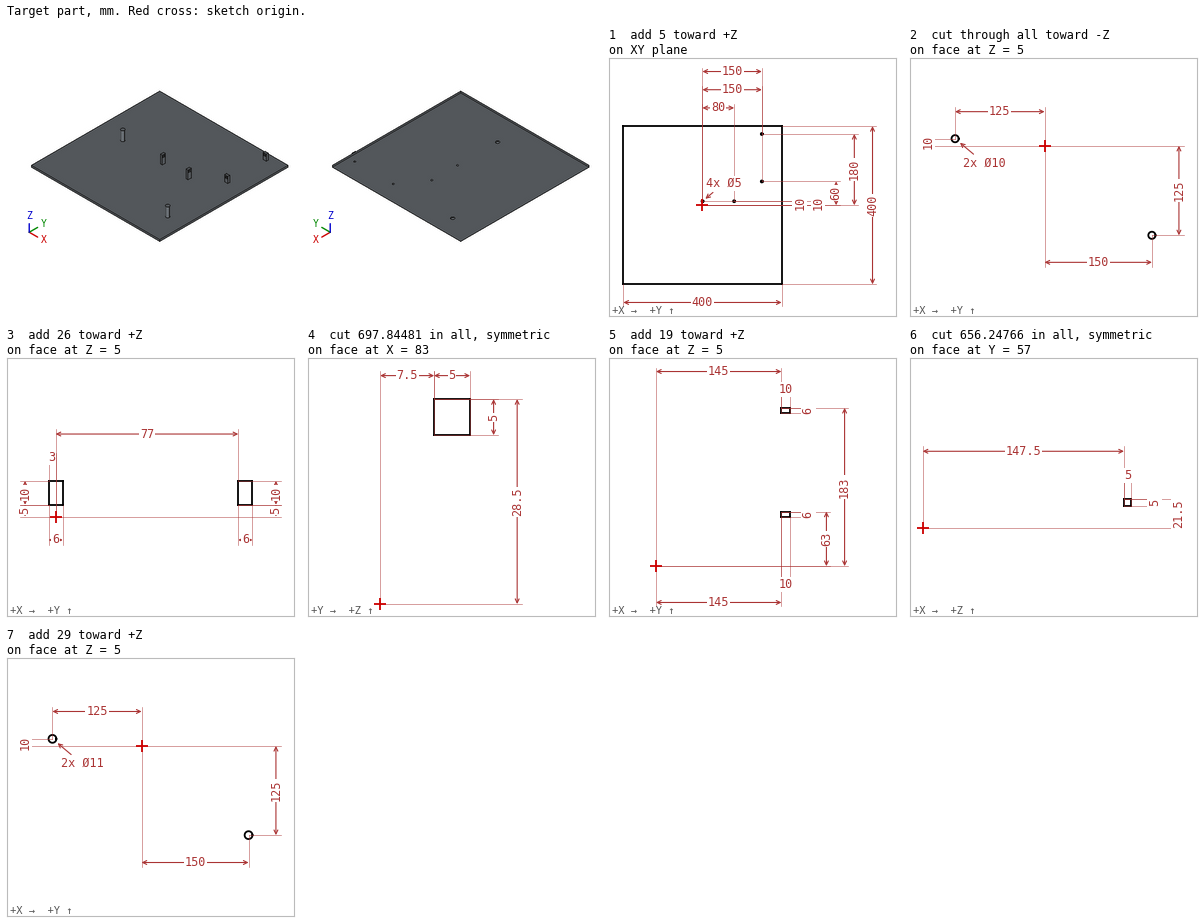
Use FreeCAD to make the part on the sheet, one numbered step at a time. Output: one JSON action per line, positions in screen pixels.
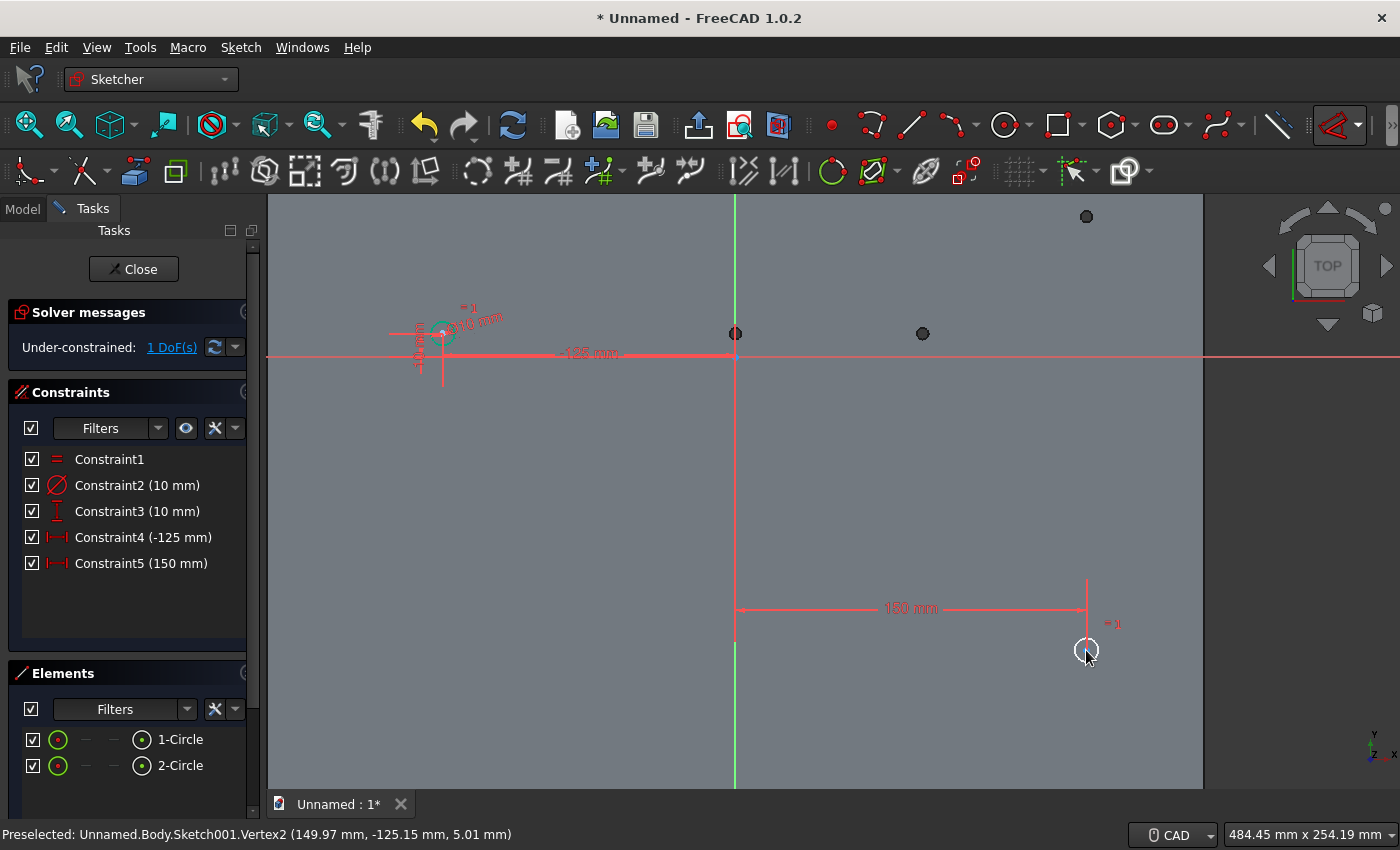
{"action": "left_click", "coordinate": [1087, 650]}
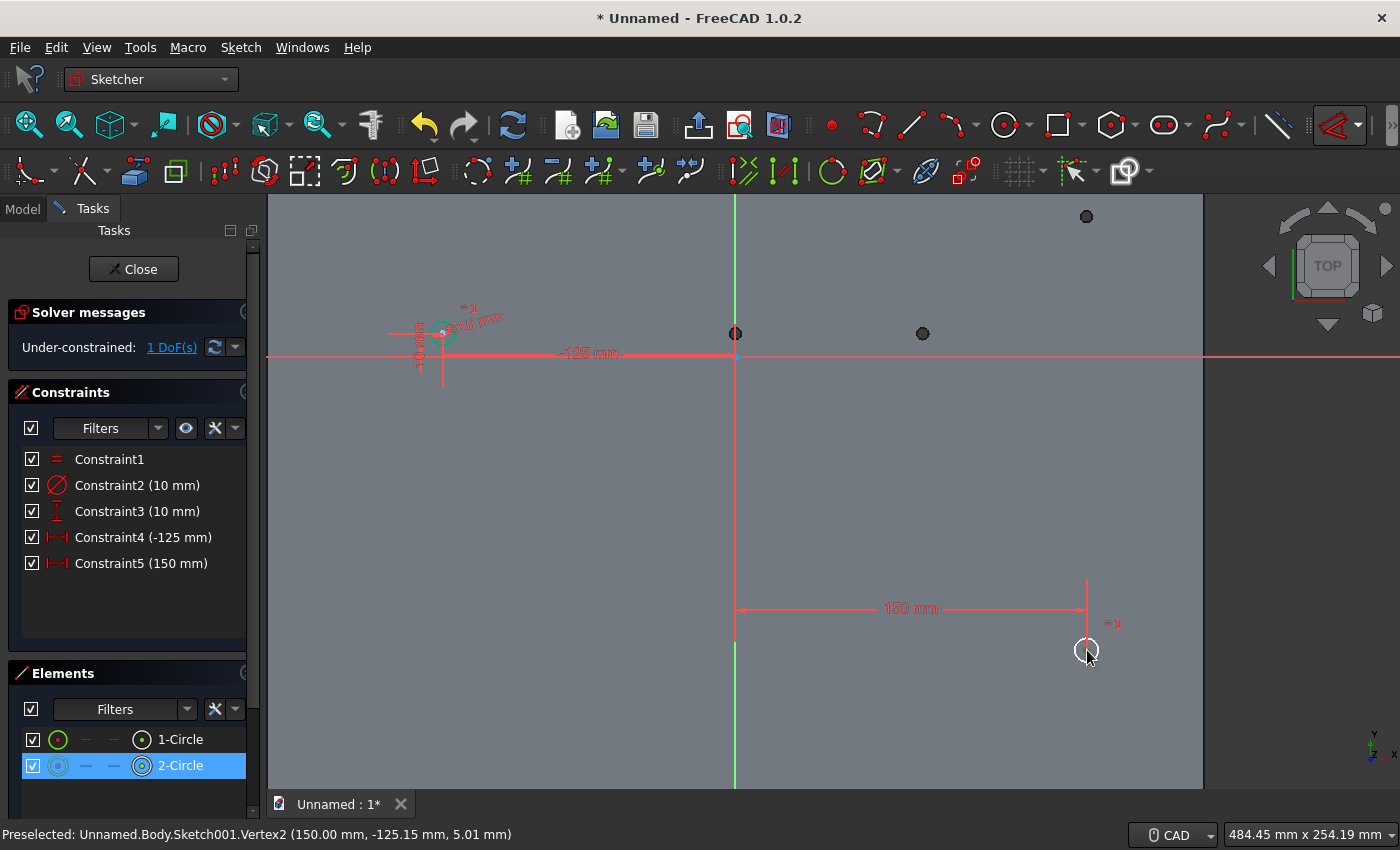
{"action": "key", "text": "i"}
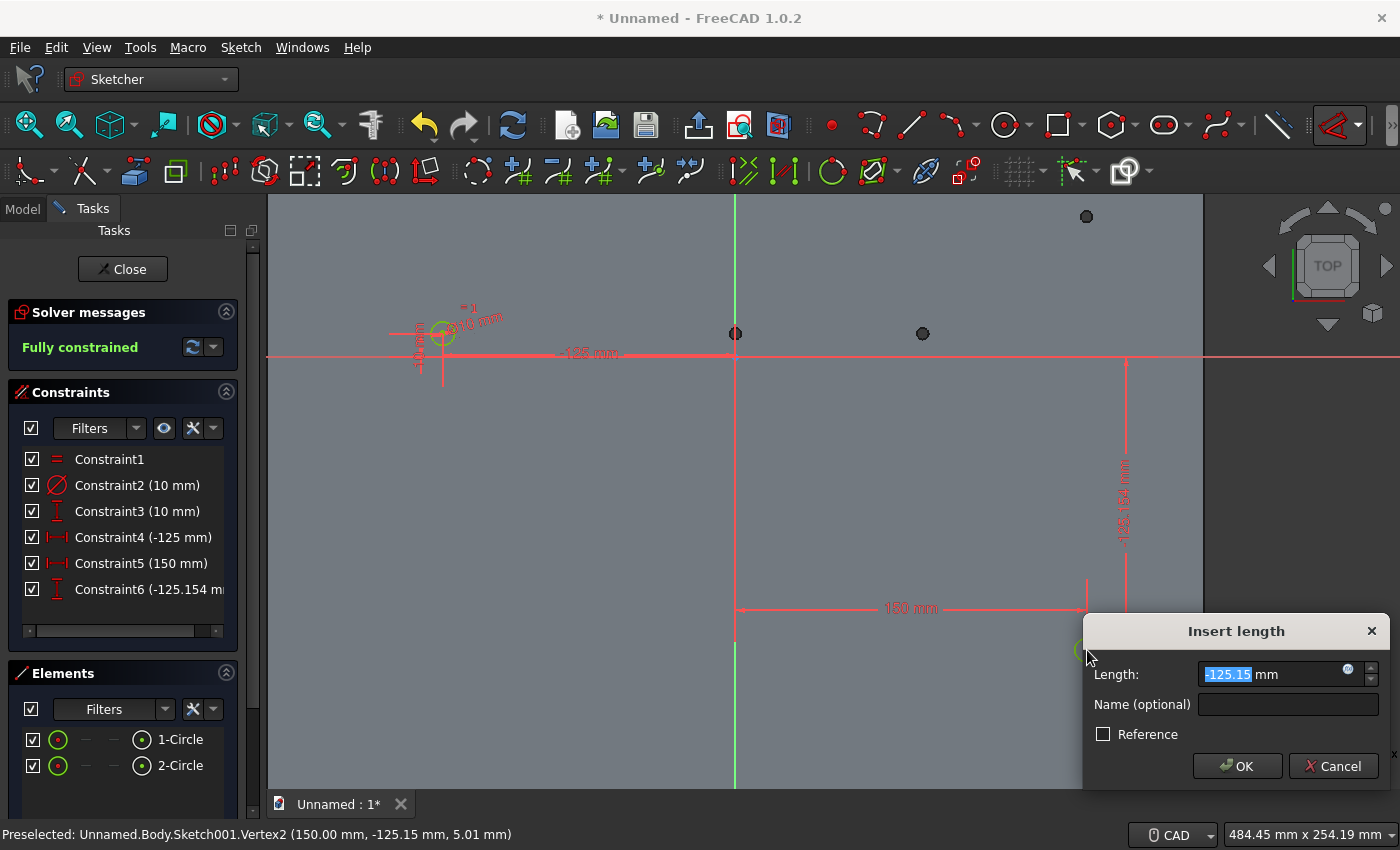
{"action": "type", "text": "-125"}
{"action": "key", "text": "Return"}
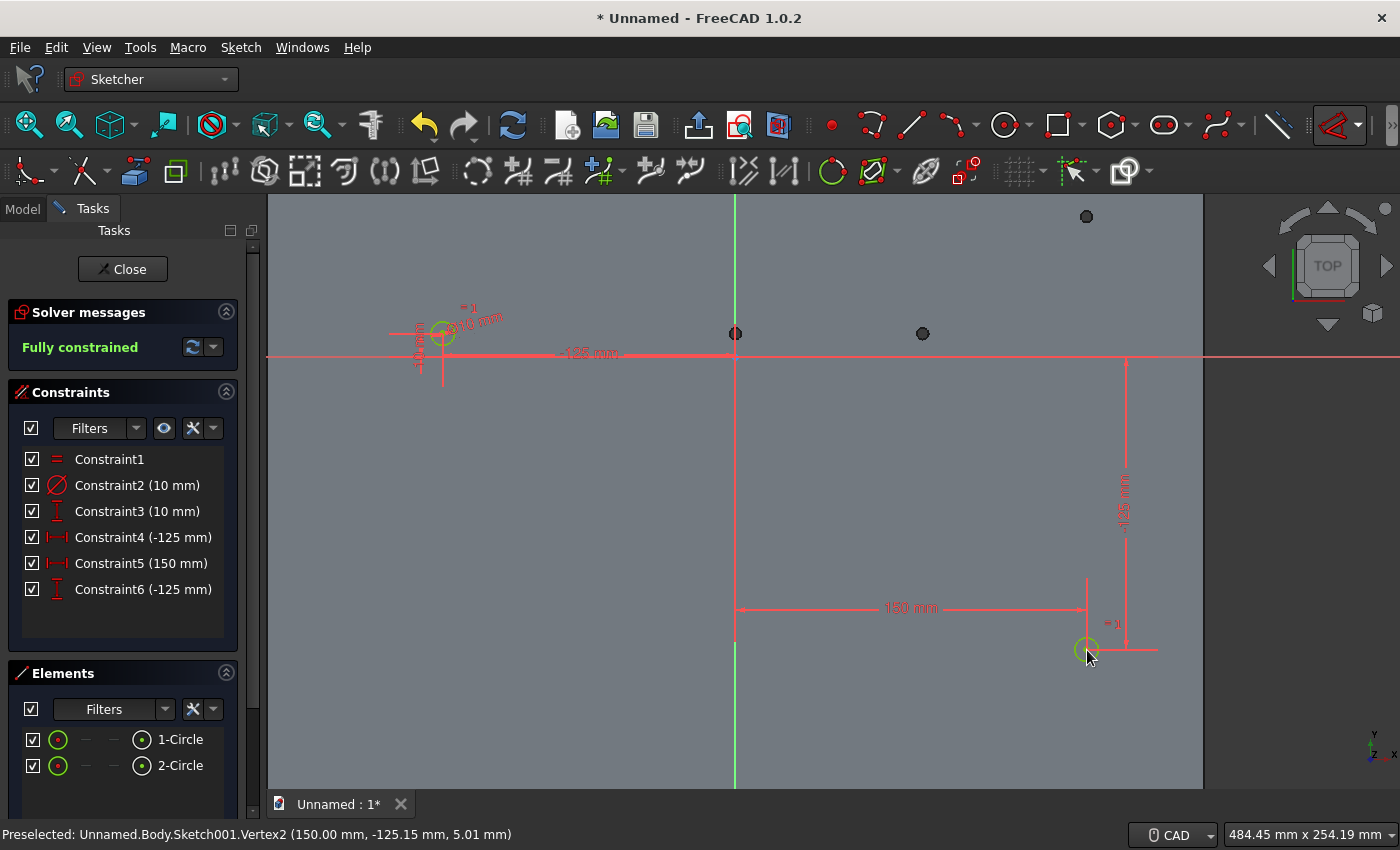
{"action": "left_click", "coordinate": [123, 269]}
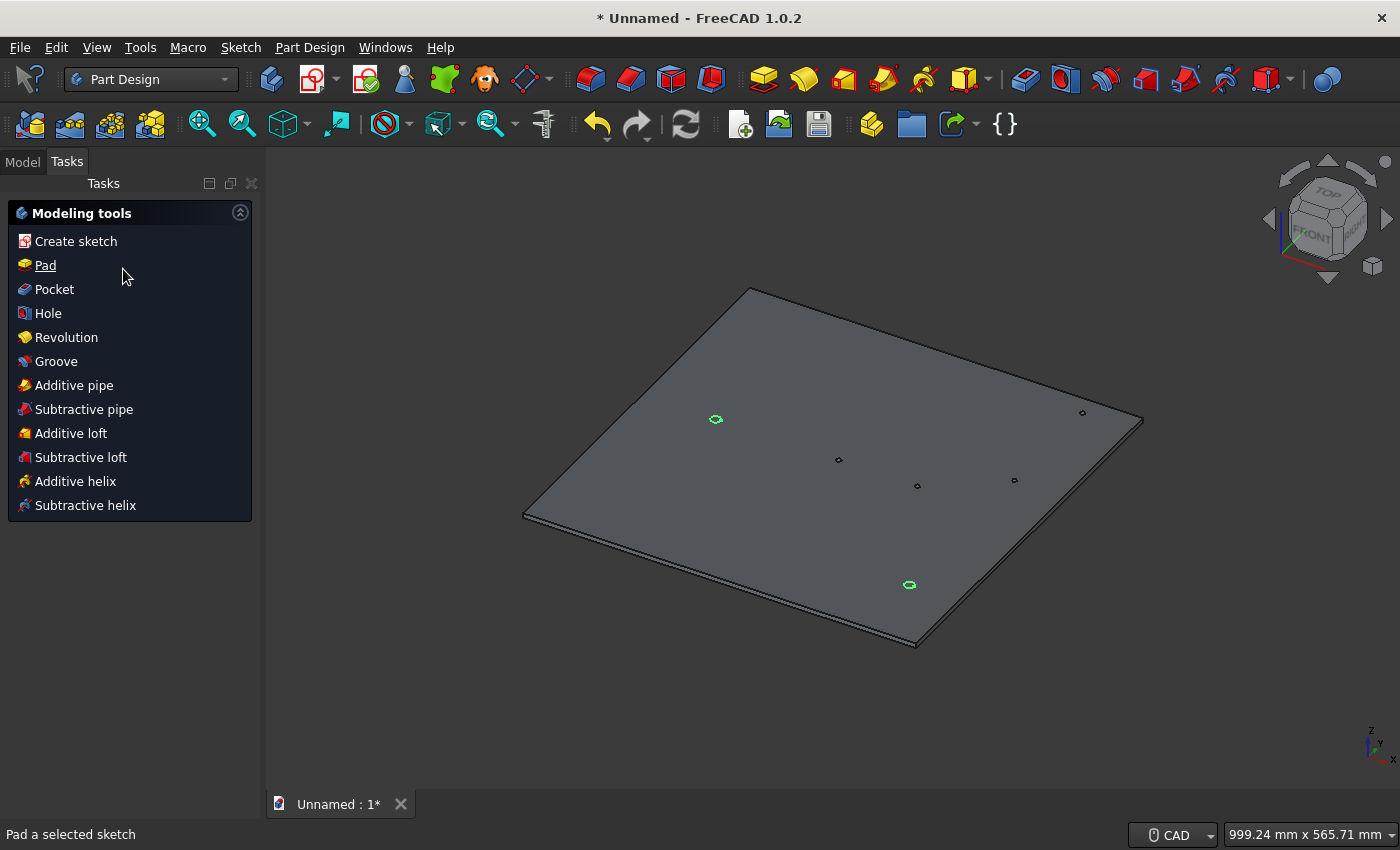
{"action": "left_click", "coordinate": [1026, 80]}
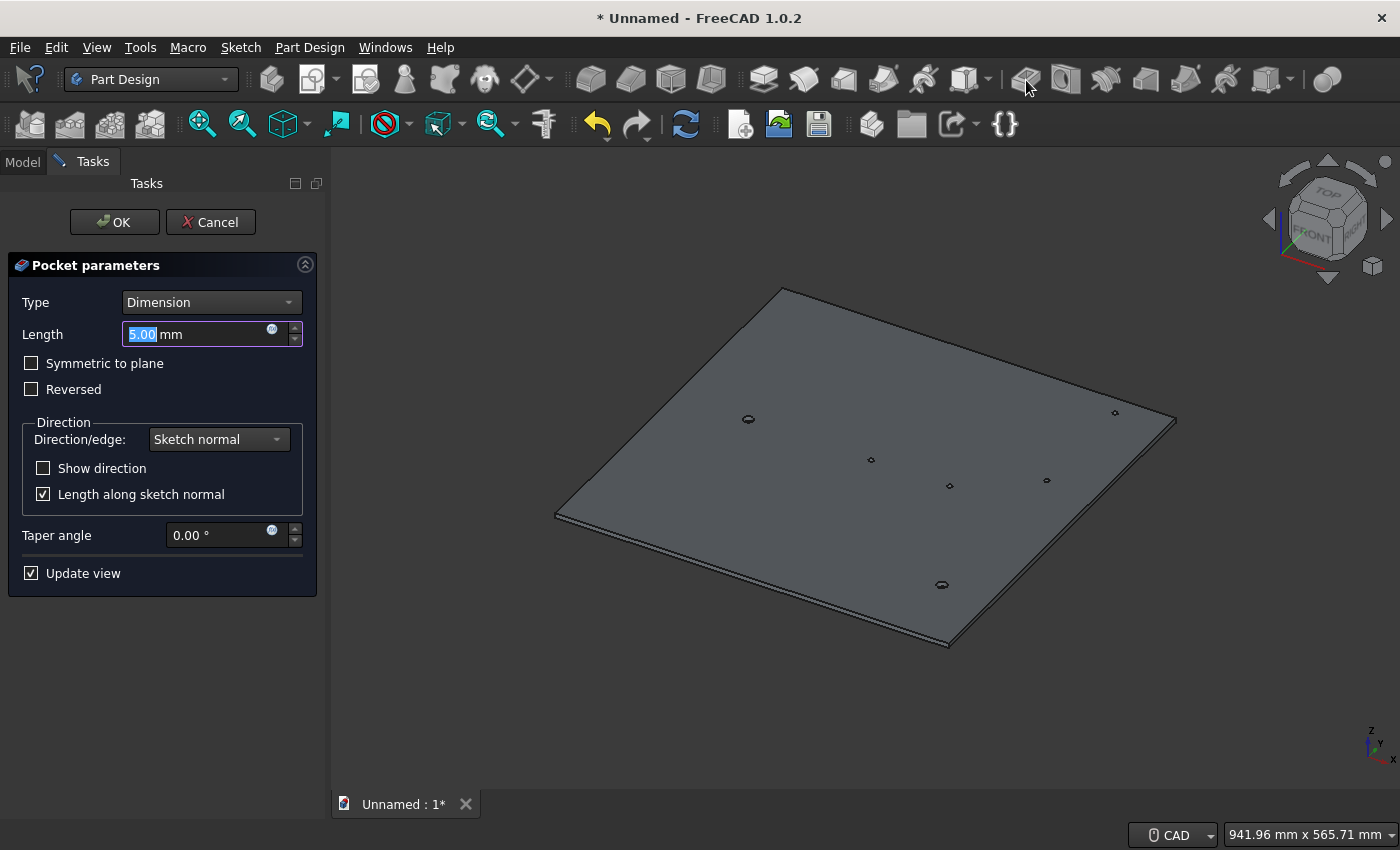
{"action": "left_click", "coordinate": [212, 302]}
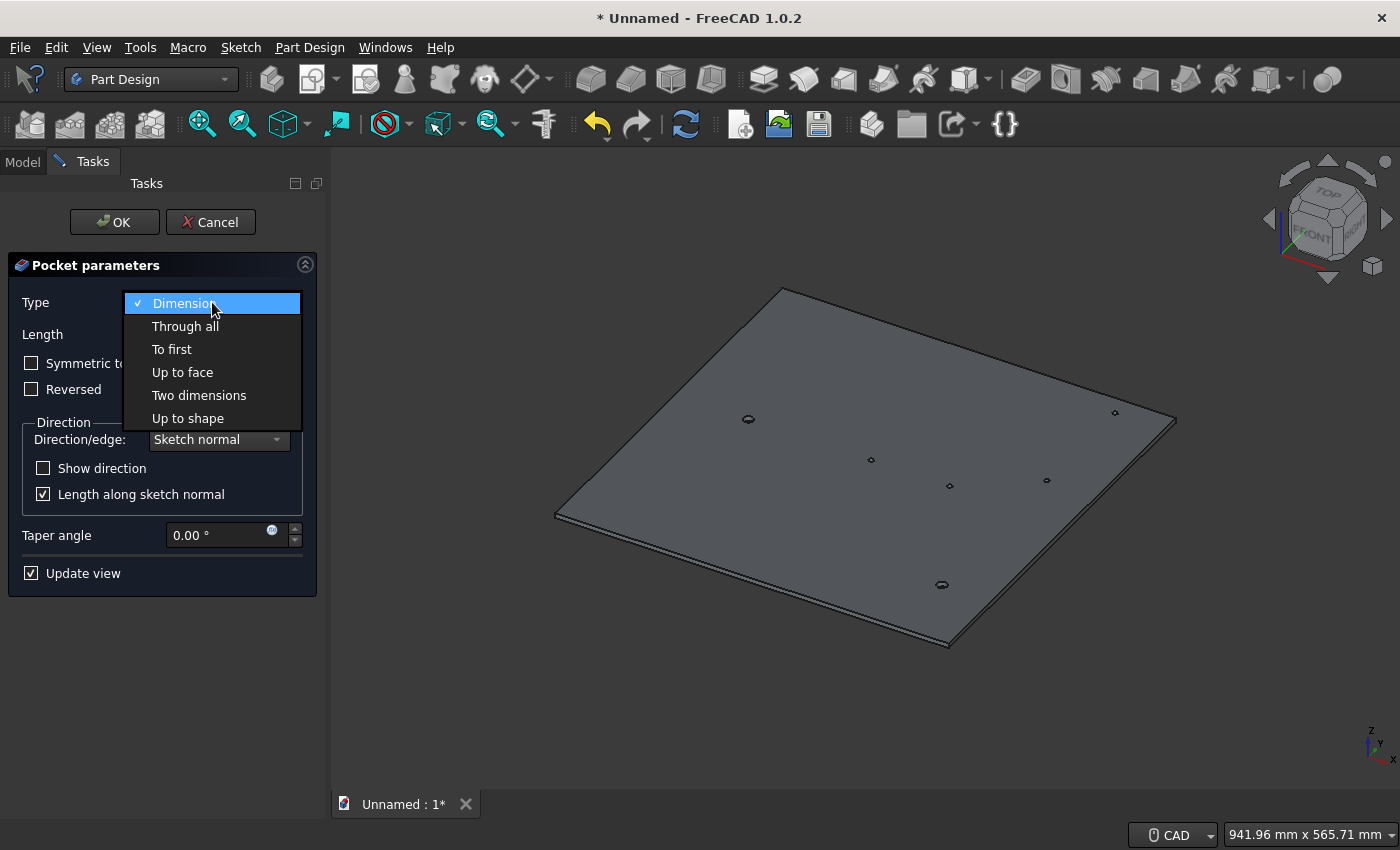
{"action": "left_click", "coordinate": [212, 326]}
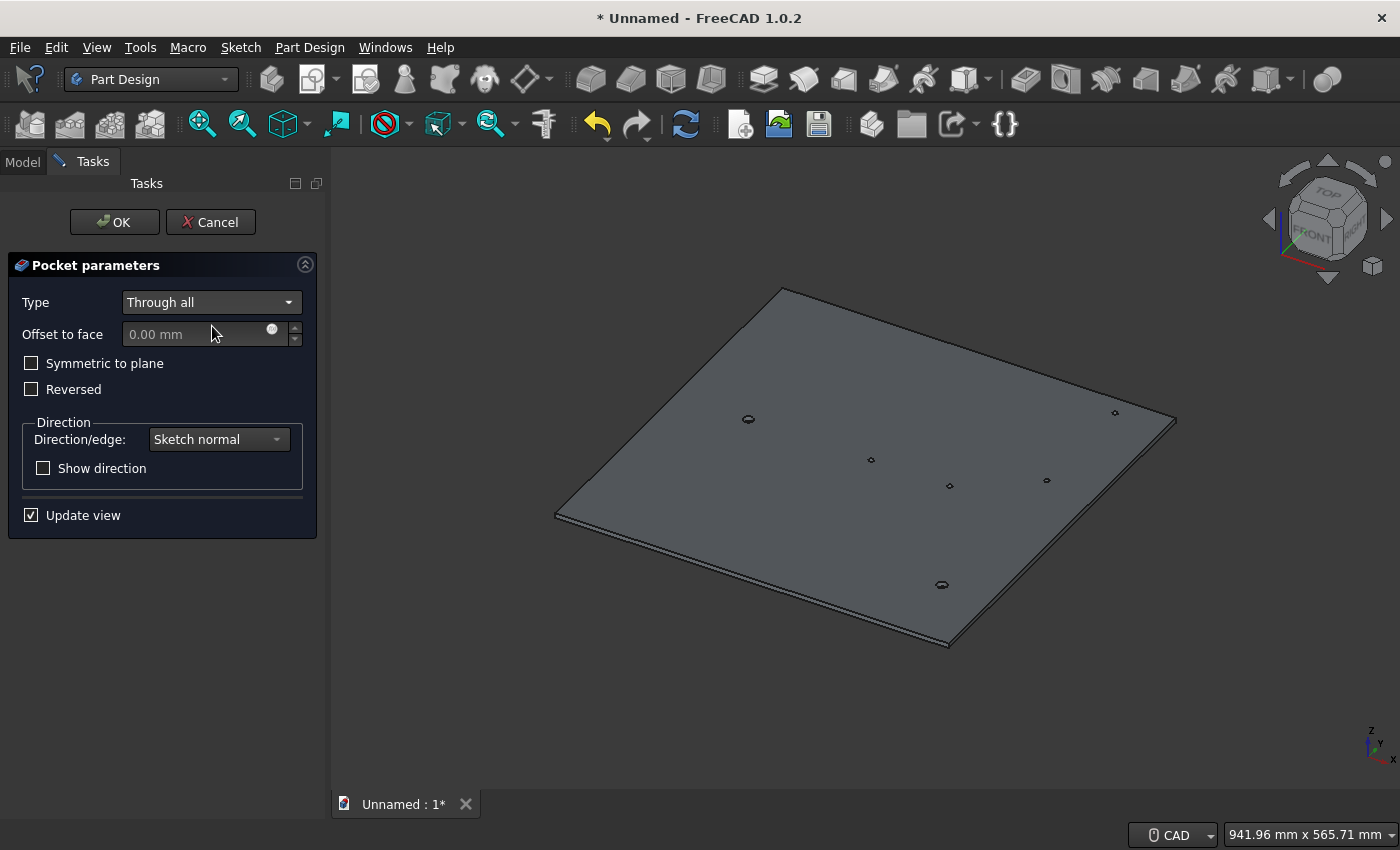
{"action": "left_click", "coordinate": [115, 222]}